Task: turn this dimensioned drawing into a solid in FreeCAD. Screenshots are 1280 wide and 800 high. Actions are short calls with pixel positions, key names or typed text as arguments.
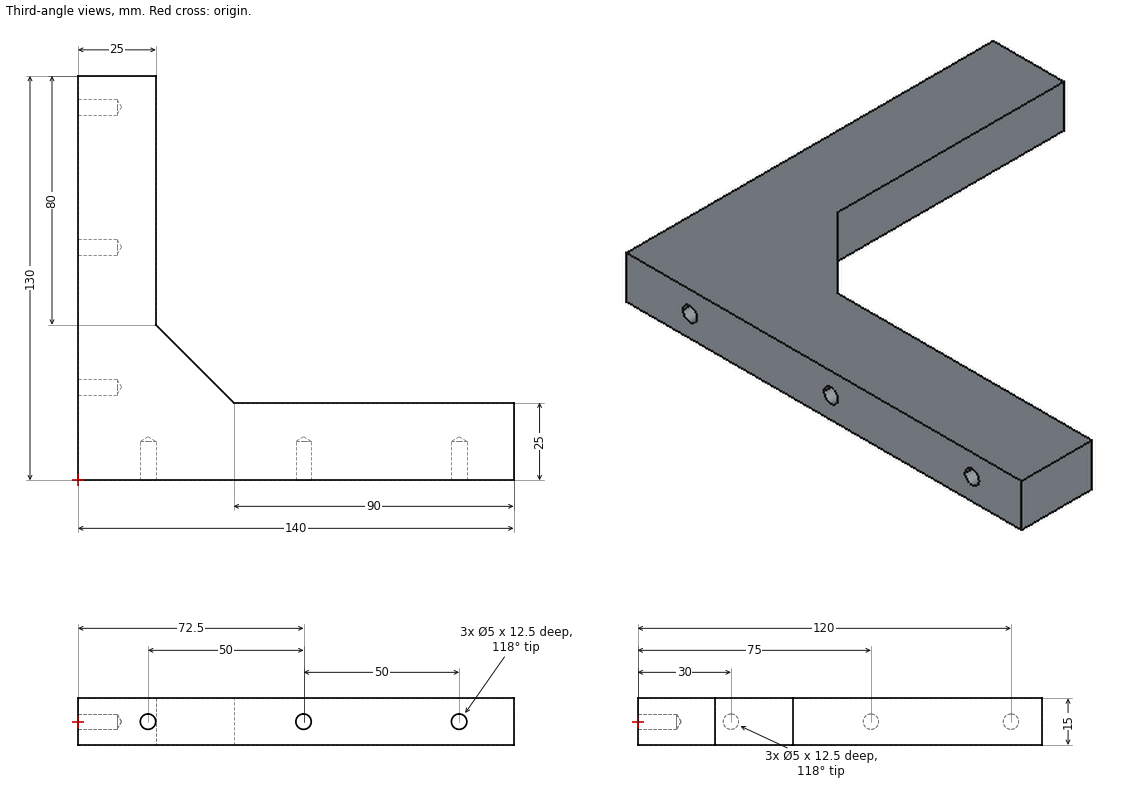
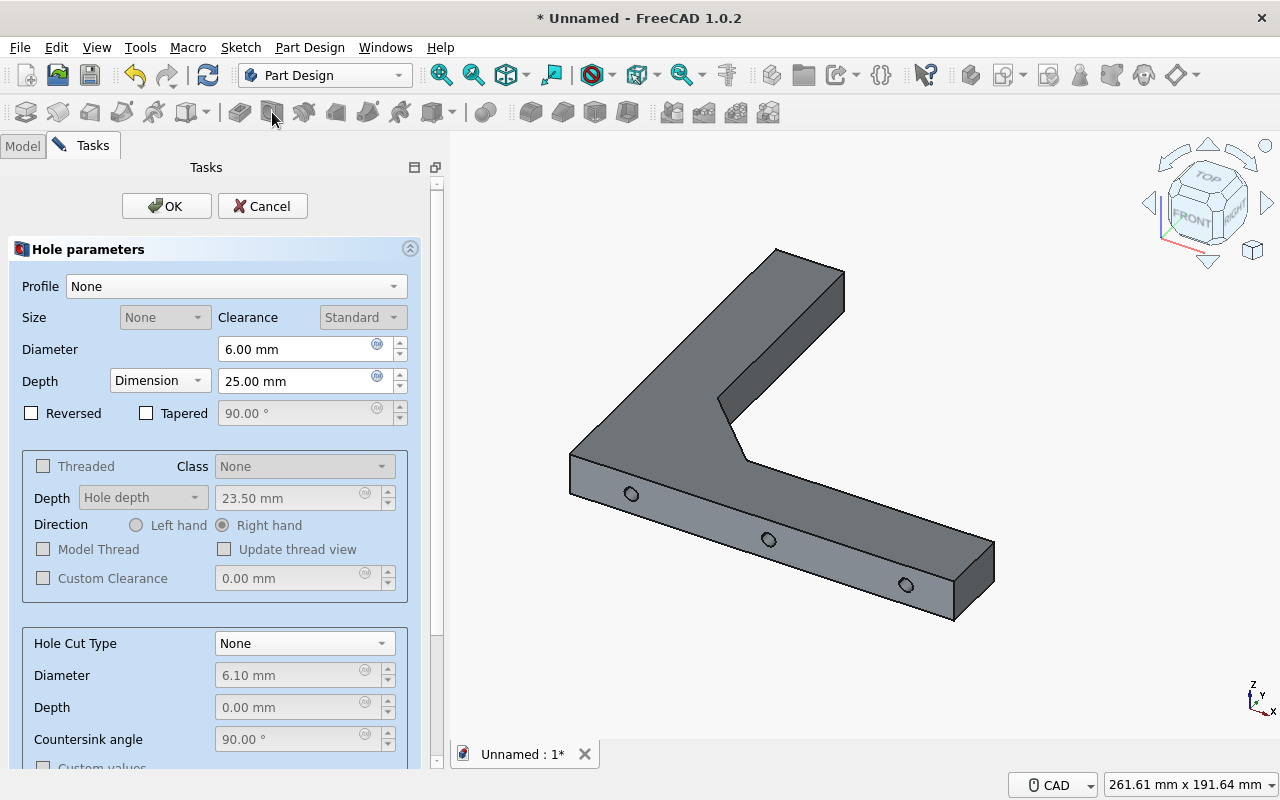
triple_click(305, 349)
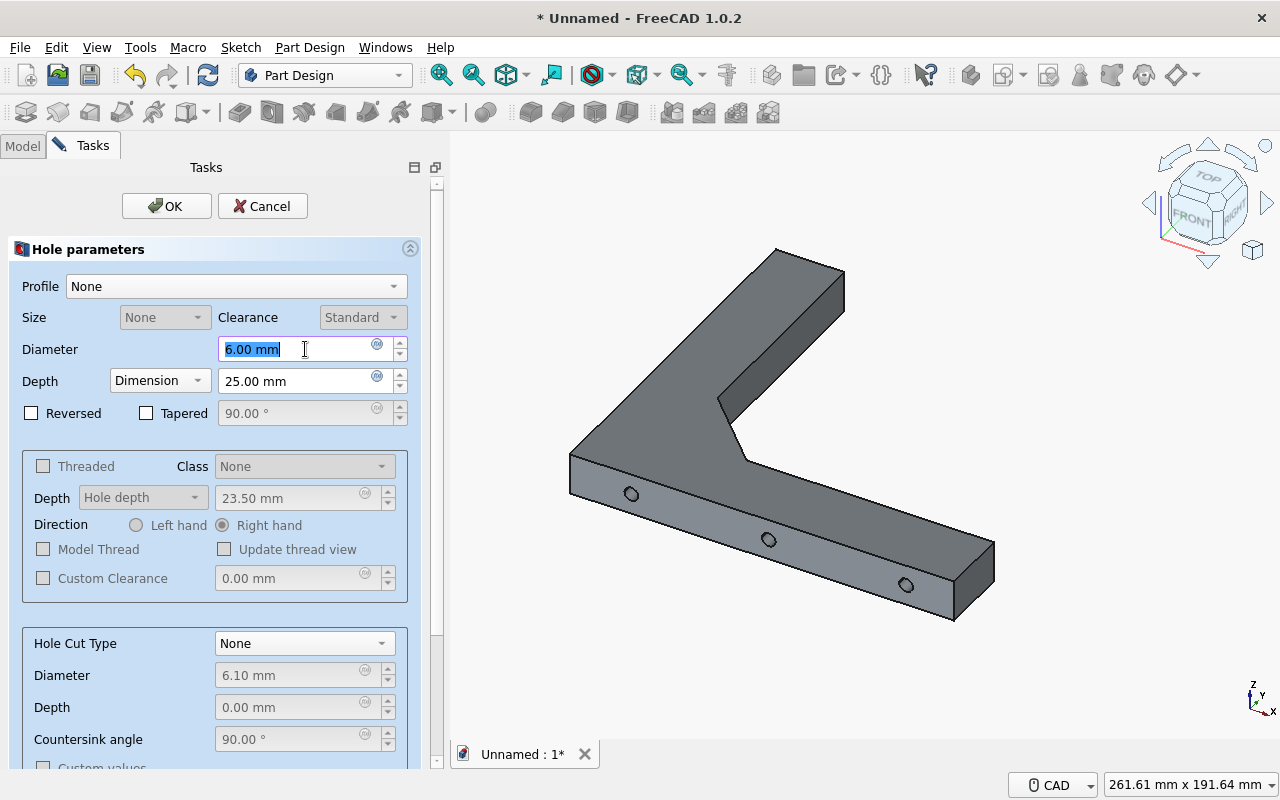
text(5)
key(Tab)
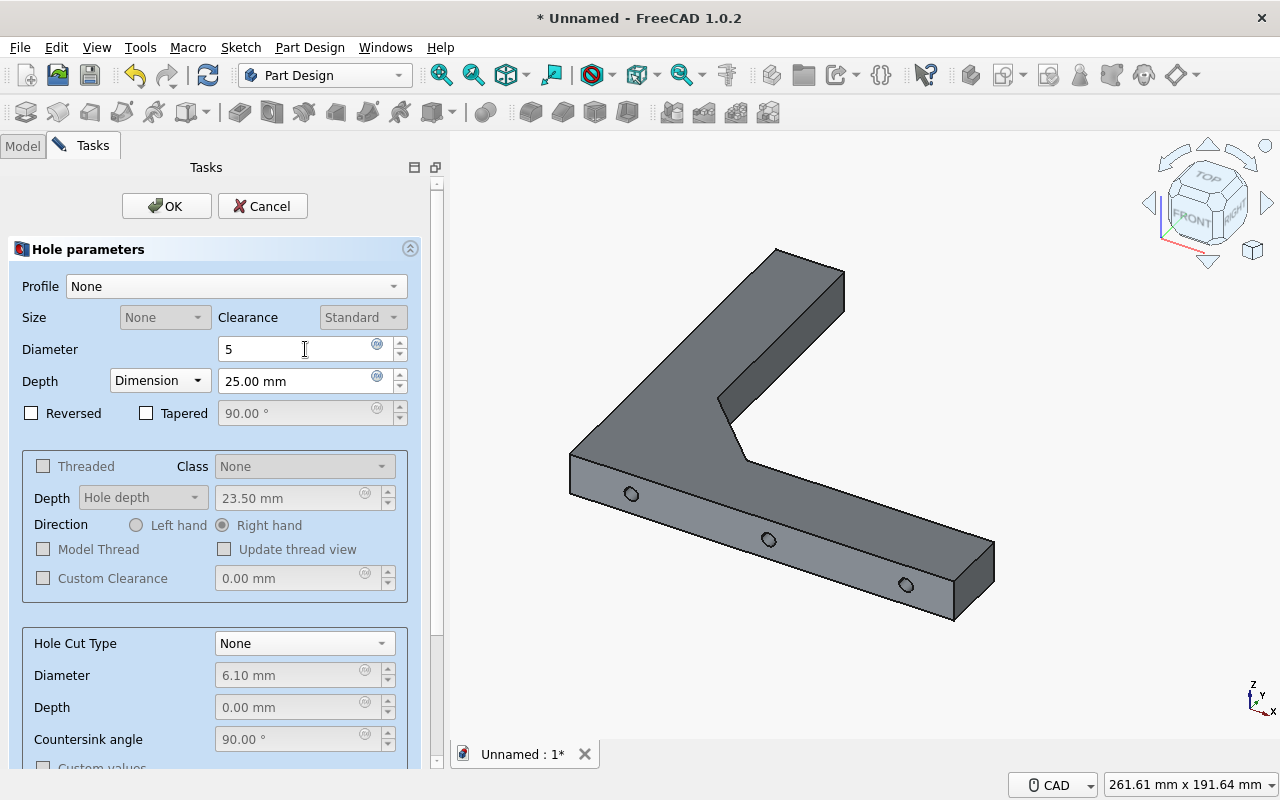
triple_click(305, 381)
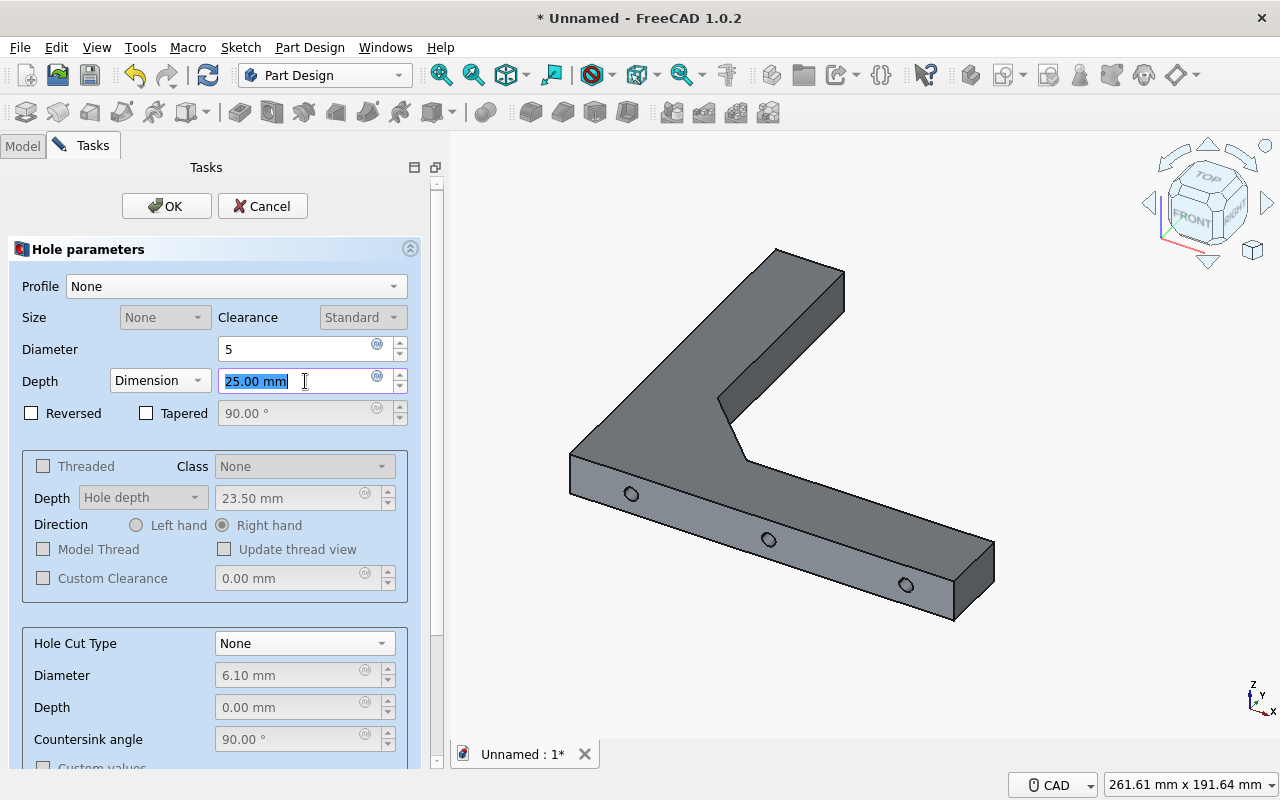
text(12.5)
key(Tab)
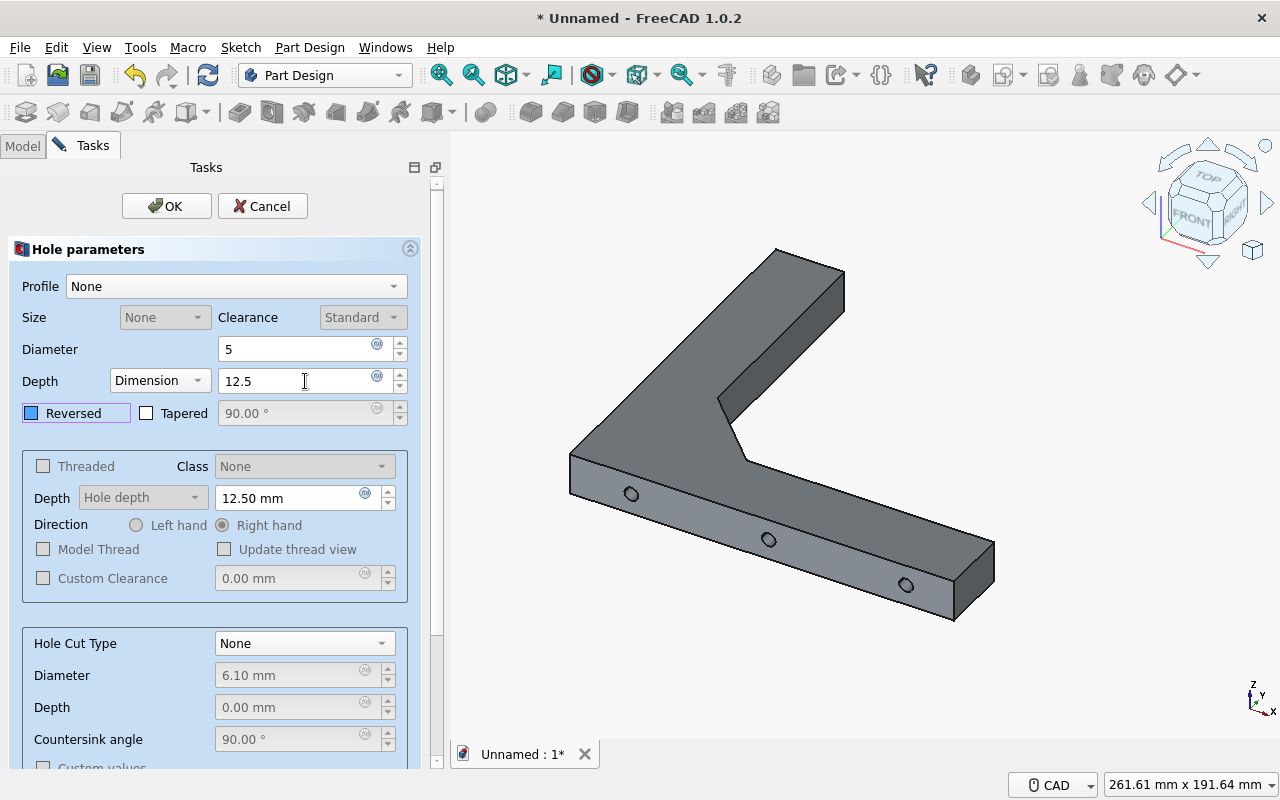
click(30, 413)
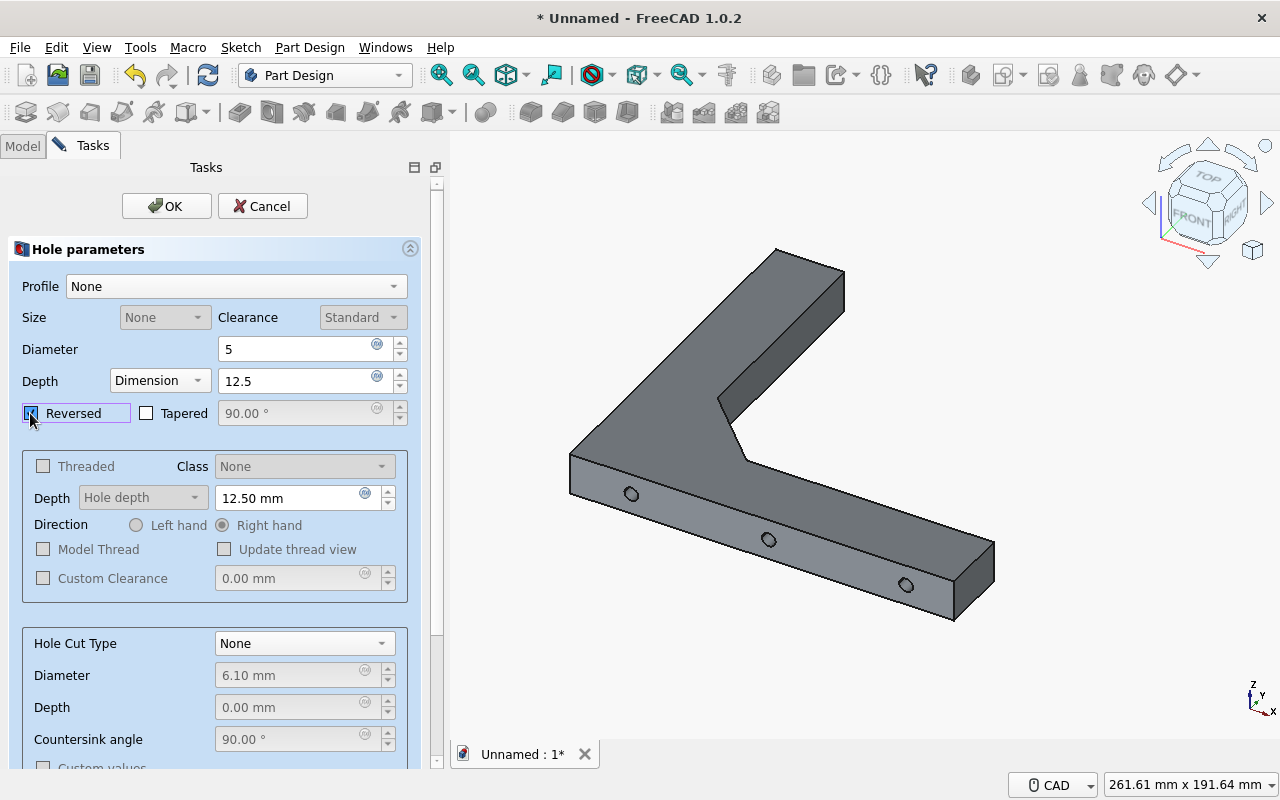
click(167, 206)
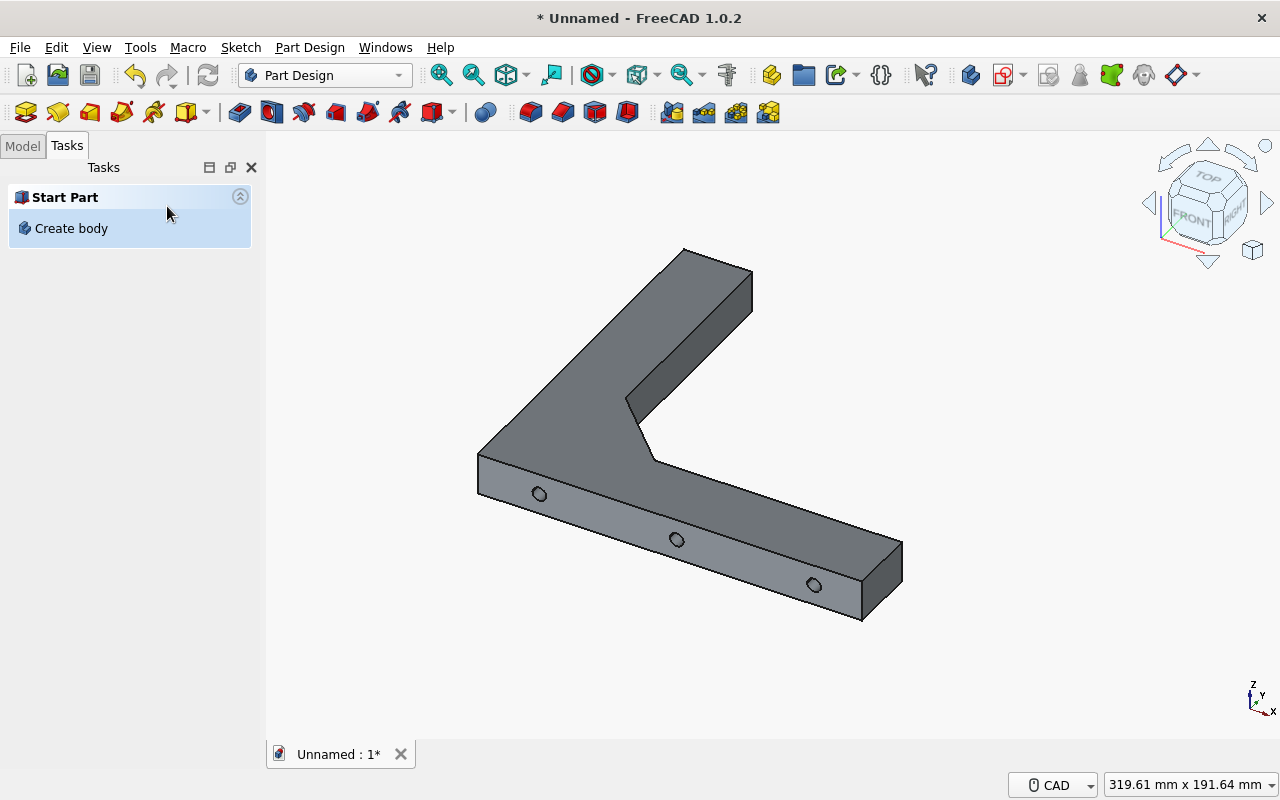
key(0)